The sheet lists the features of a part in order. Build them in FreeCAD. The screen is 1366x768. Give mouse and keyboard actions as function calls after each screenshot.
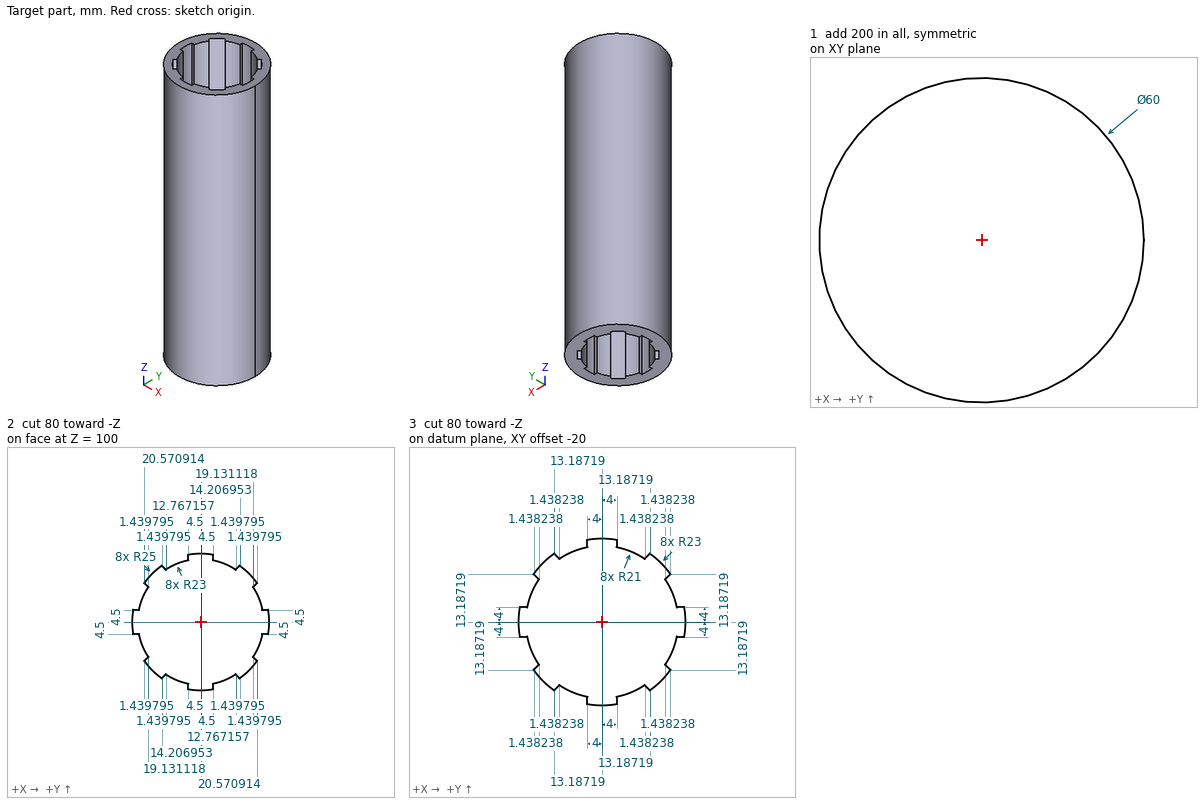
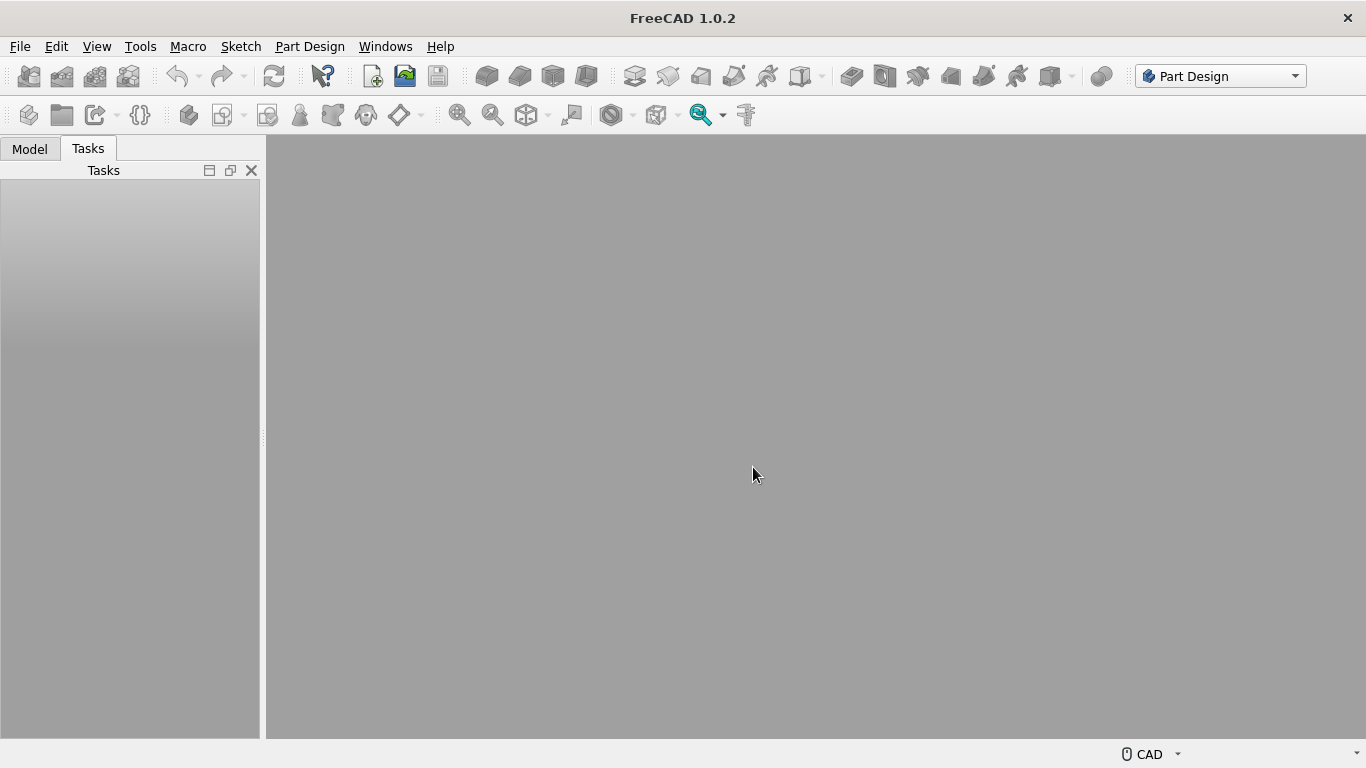
click(372, 76)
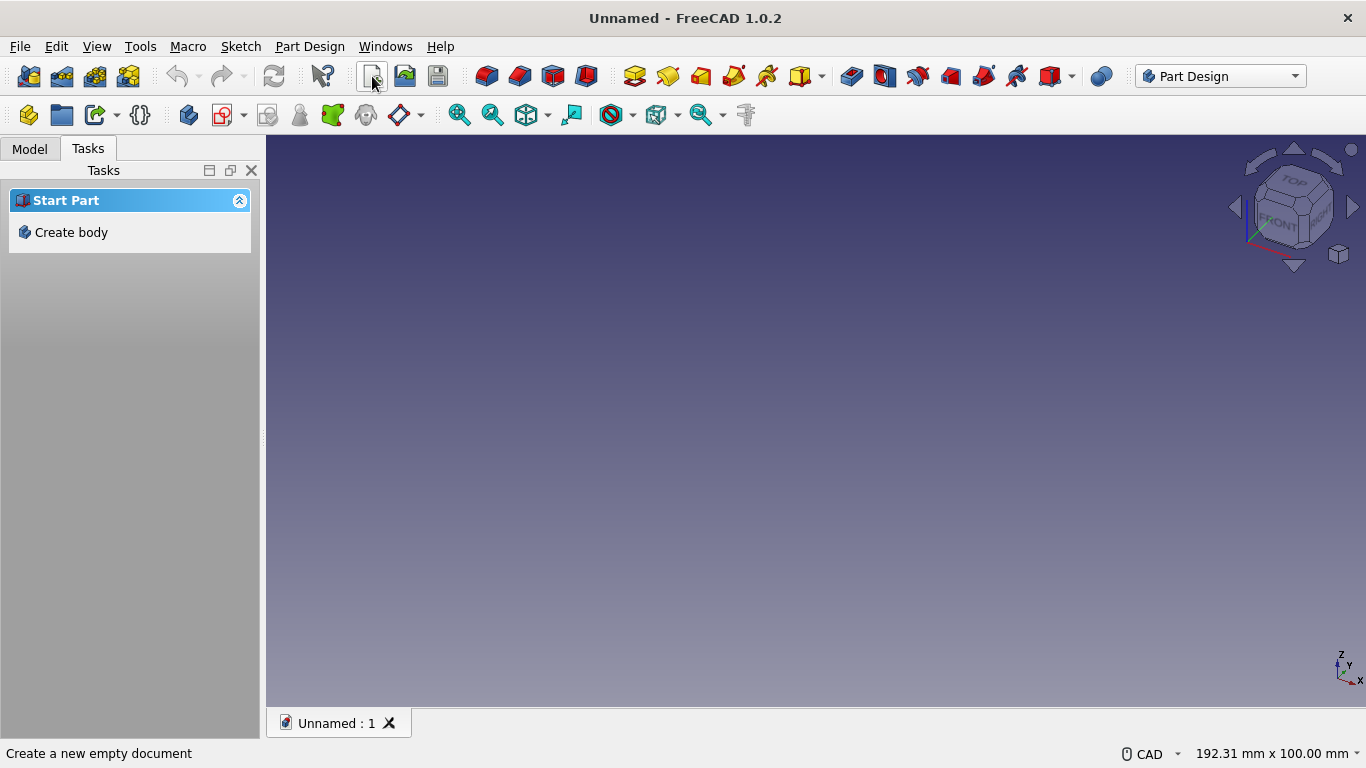
click(222, 116)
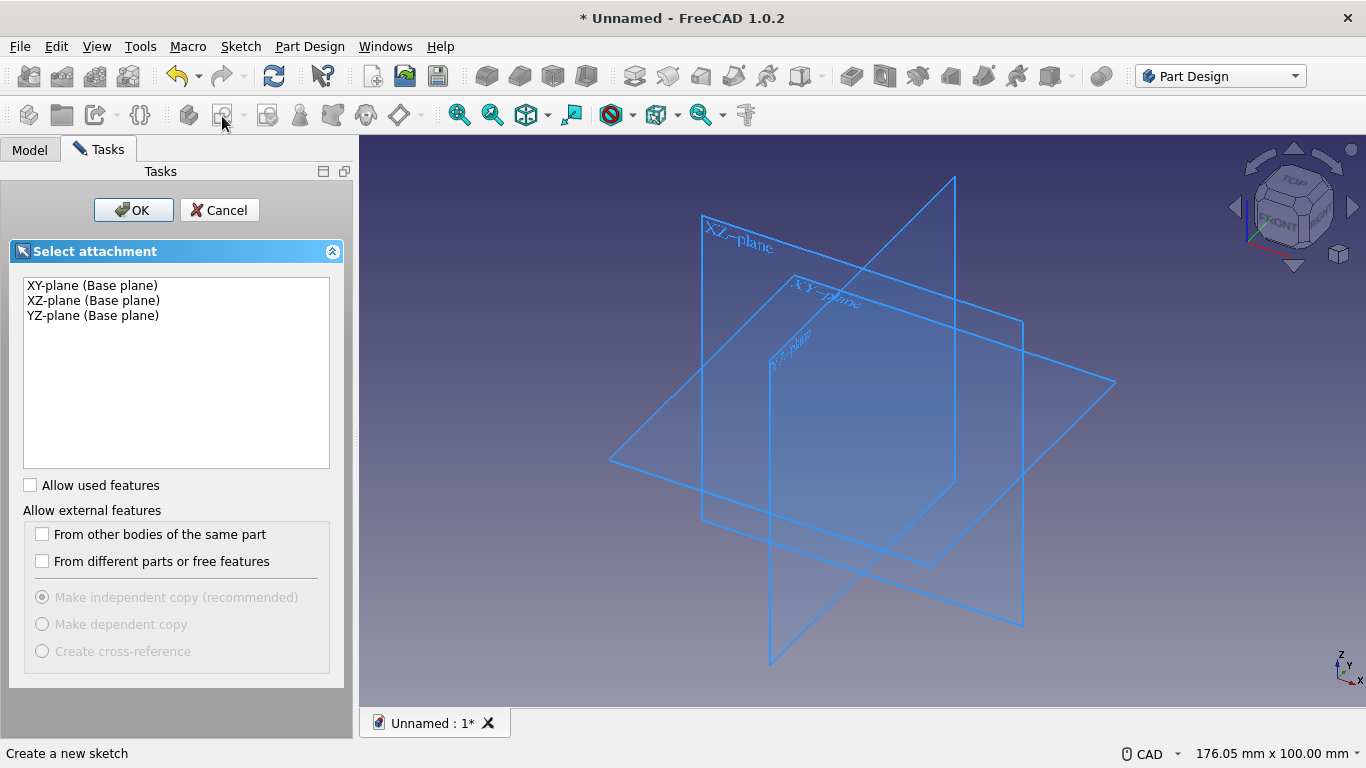
click(84, 286)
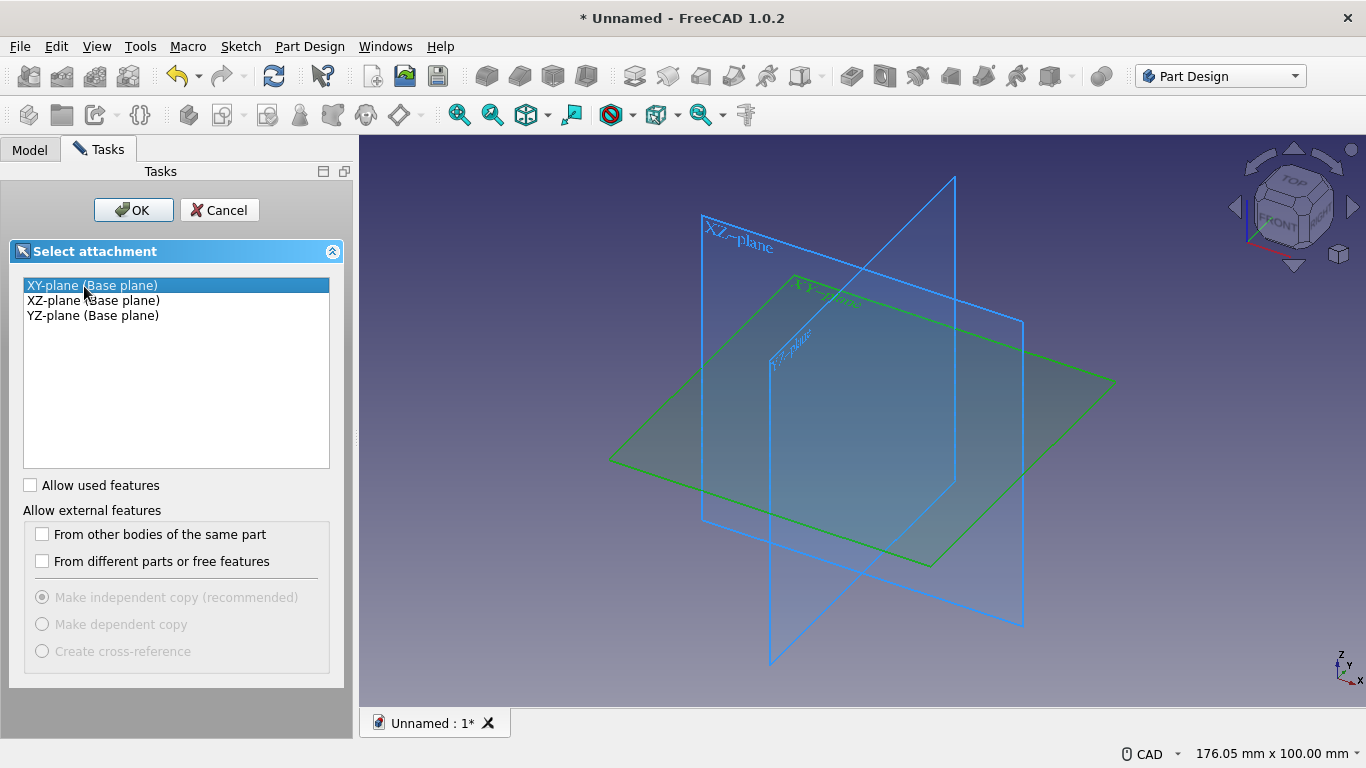
click(134, 210)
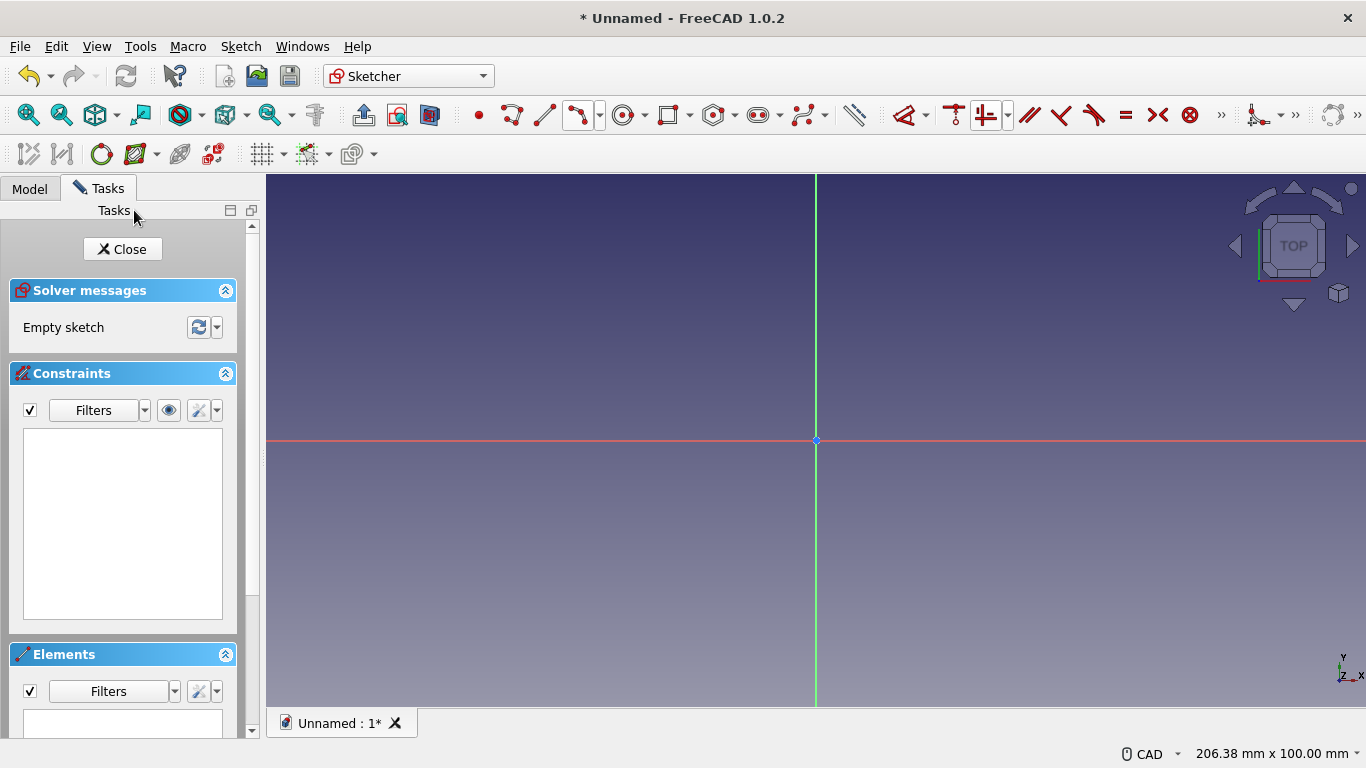
click(622, 116)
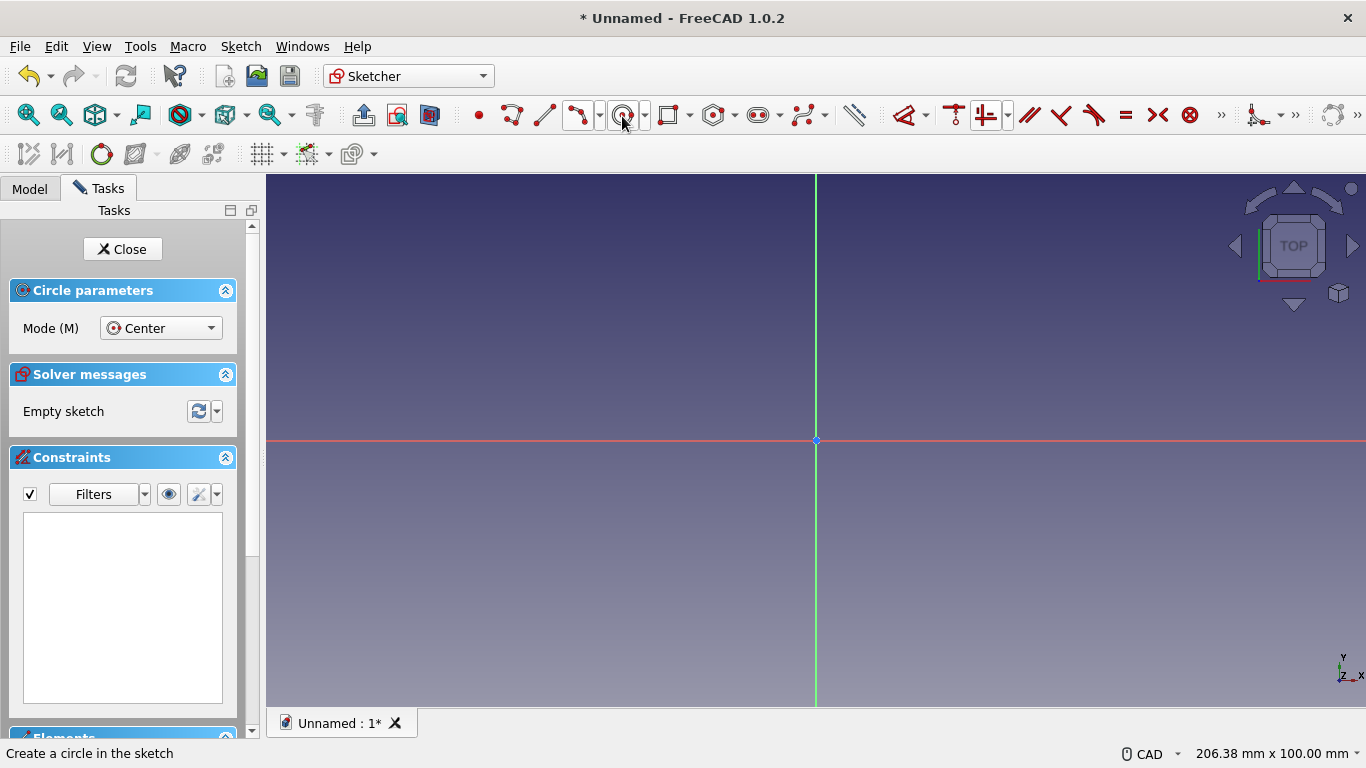
click(816, 440)
move(929, 327)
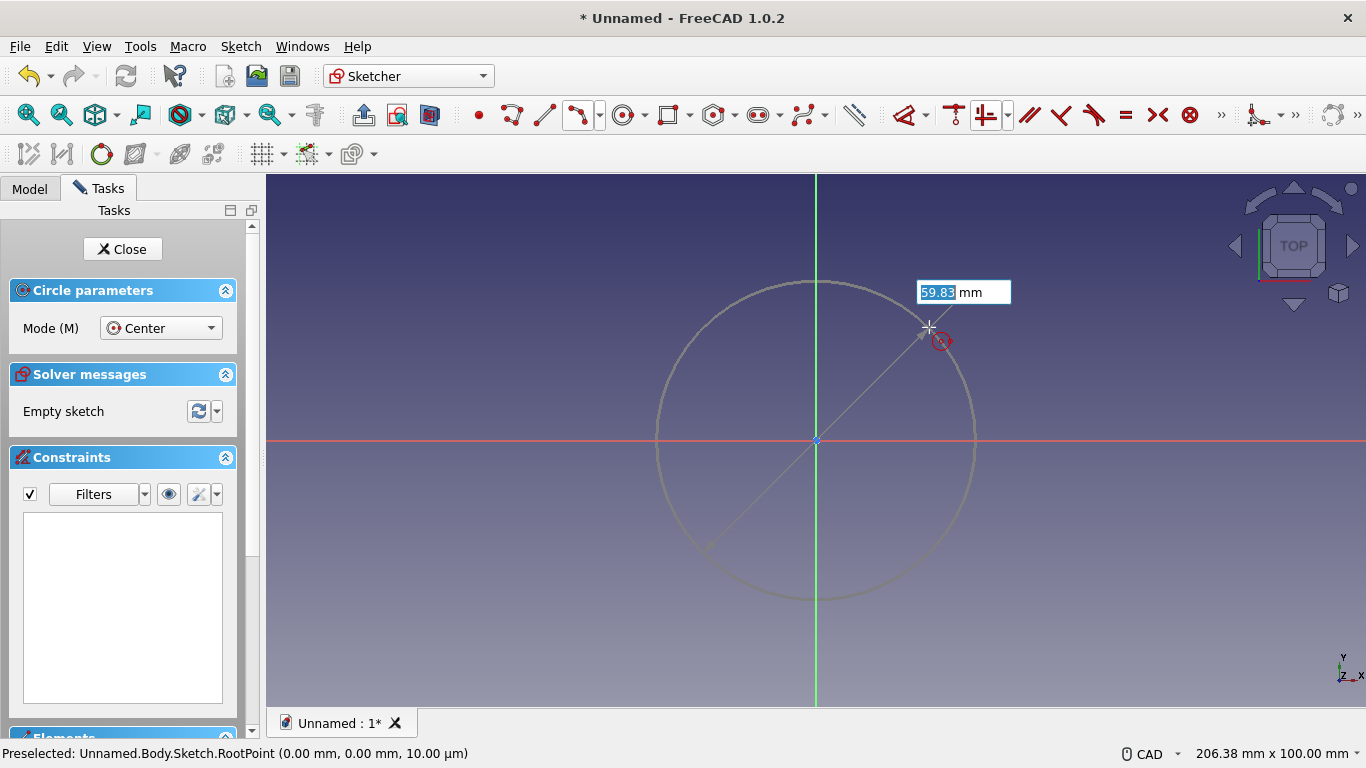
text(60)
key(Return)
key(Escape)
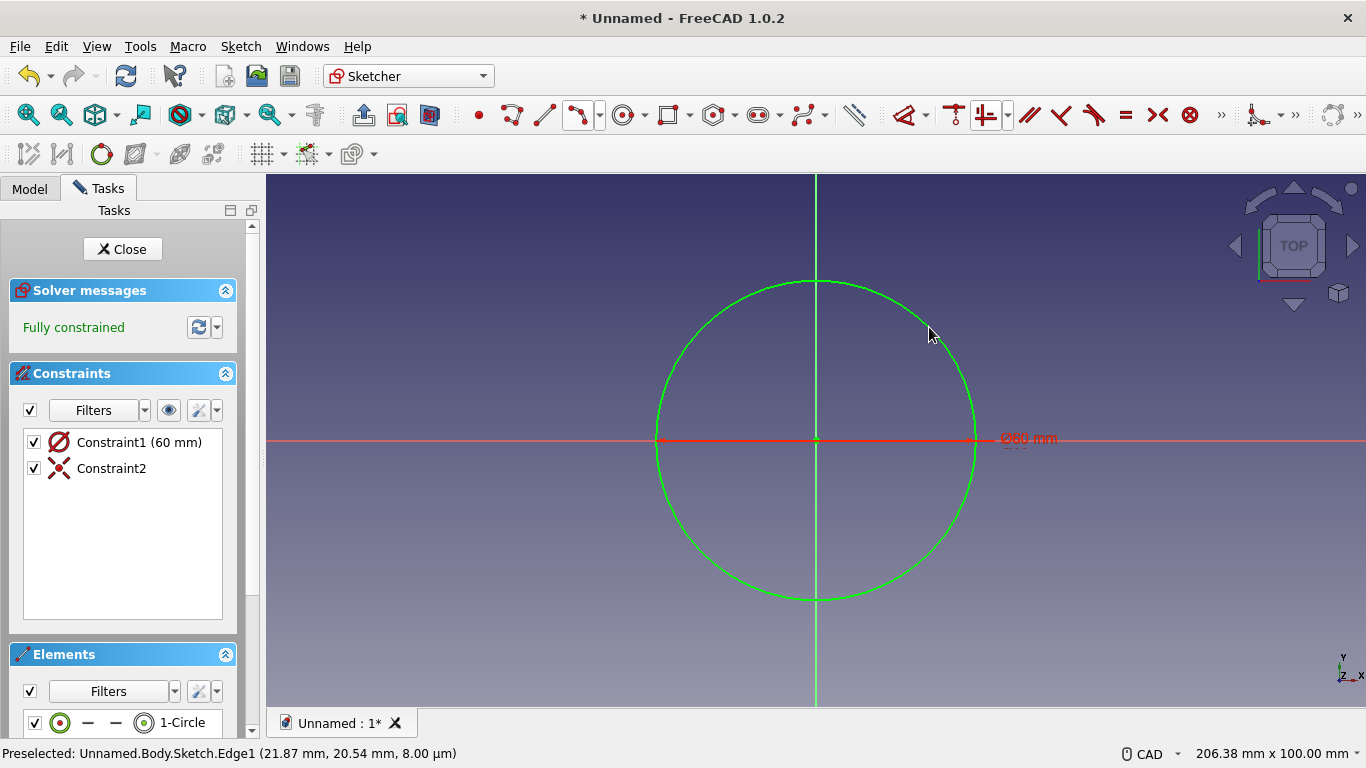
click(123, 249)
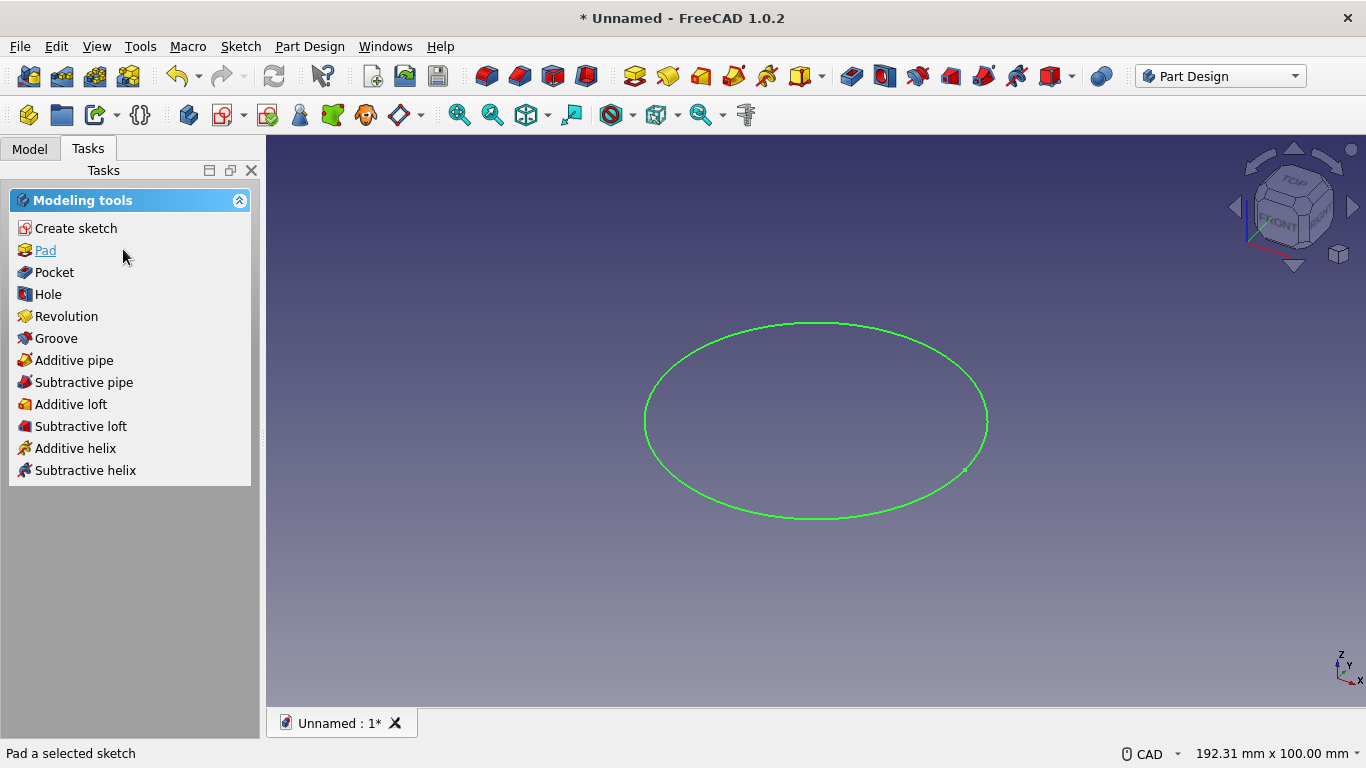
click(635, 76)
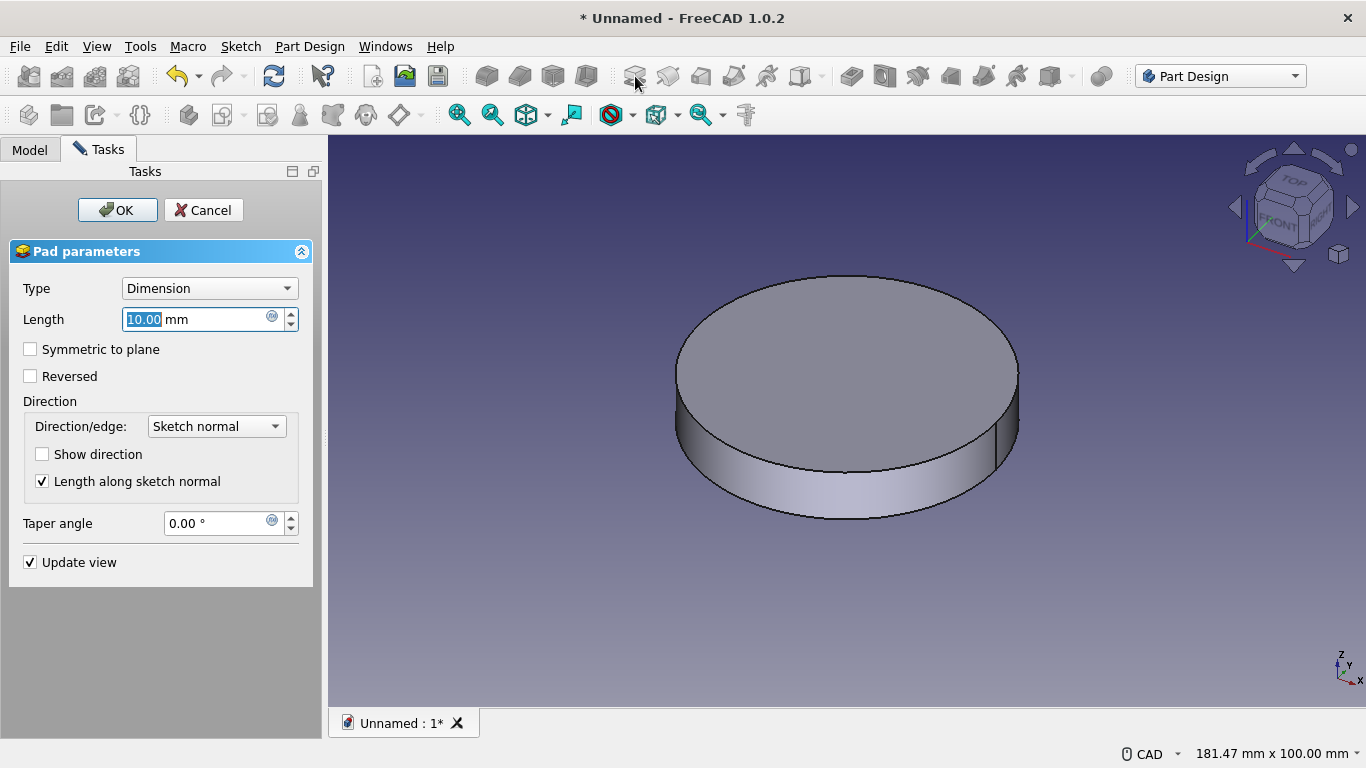
text(200)
key(Tab)